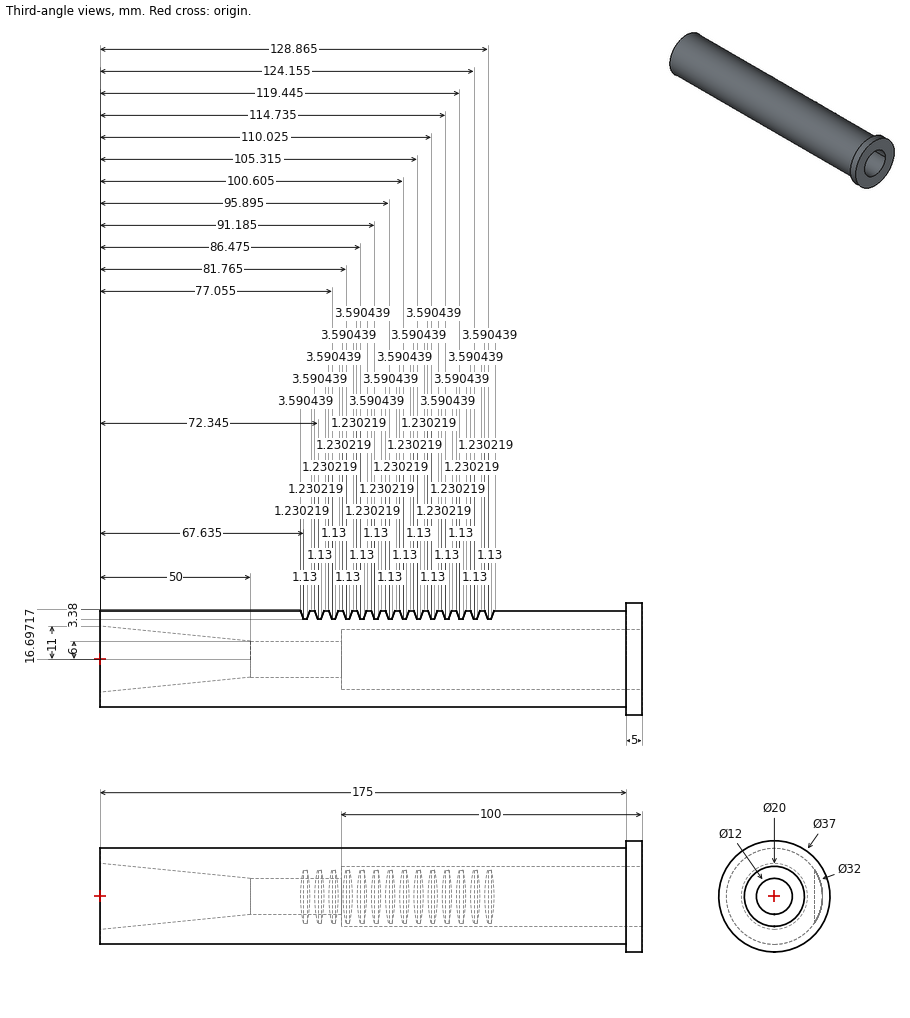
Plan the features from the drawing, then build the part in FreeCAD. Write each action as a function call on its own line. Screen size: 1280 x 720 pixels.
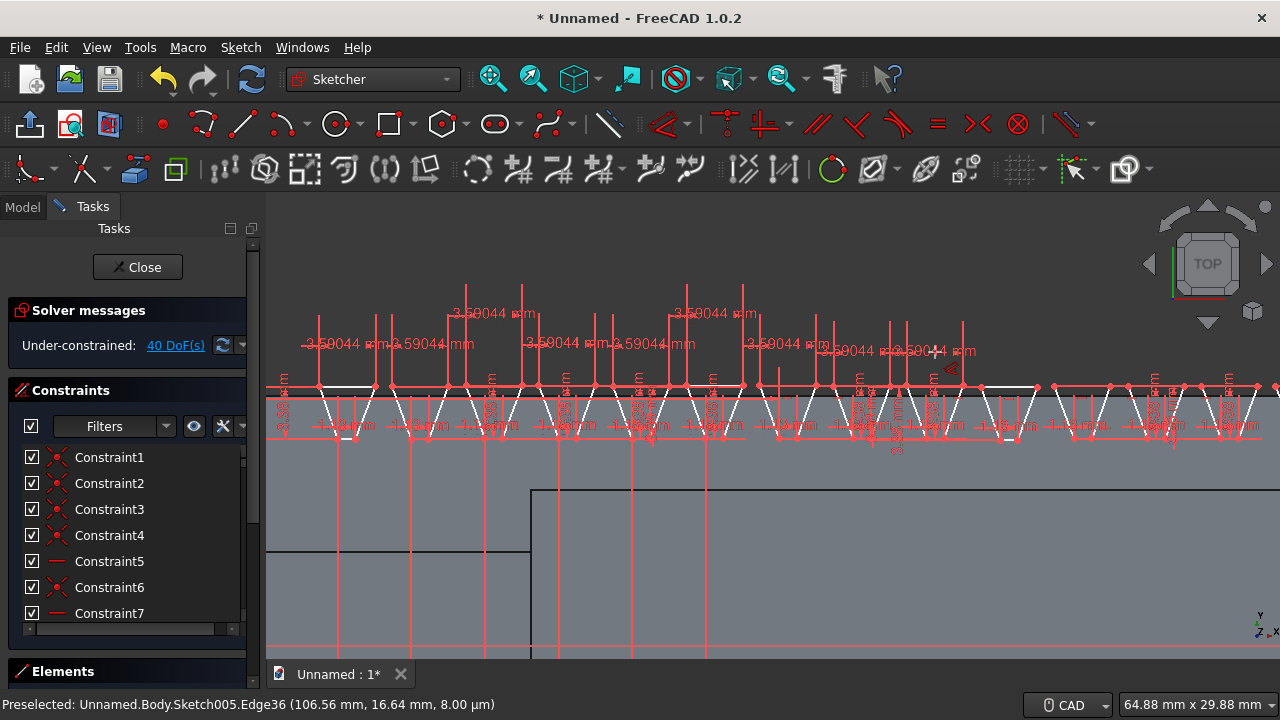
click(1020, 387)
click(1009, 353)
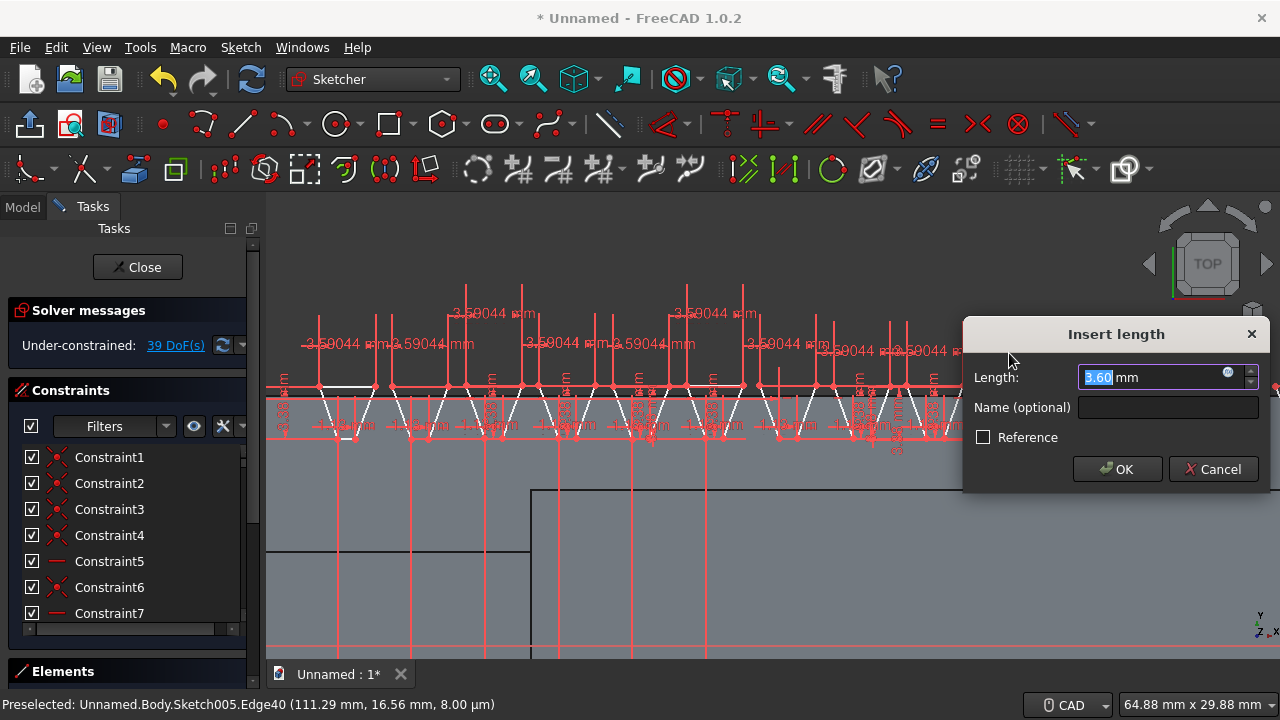
text(3.590439)
key(Return)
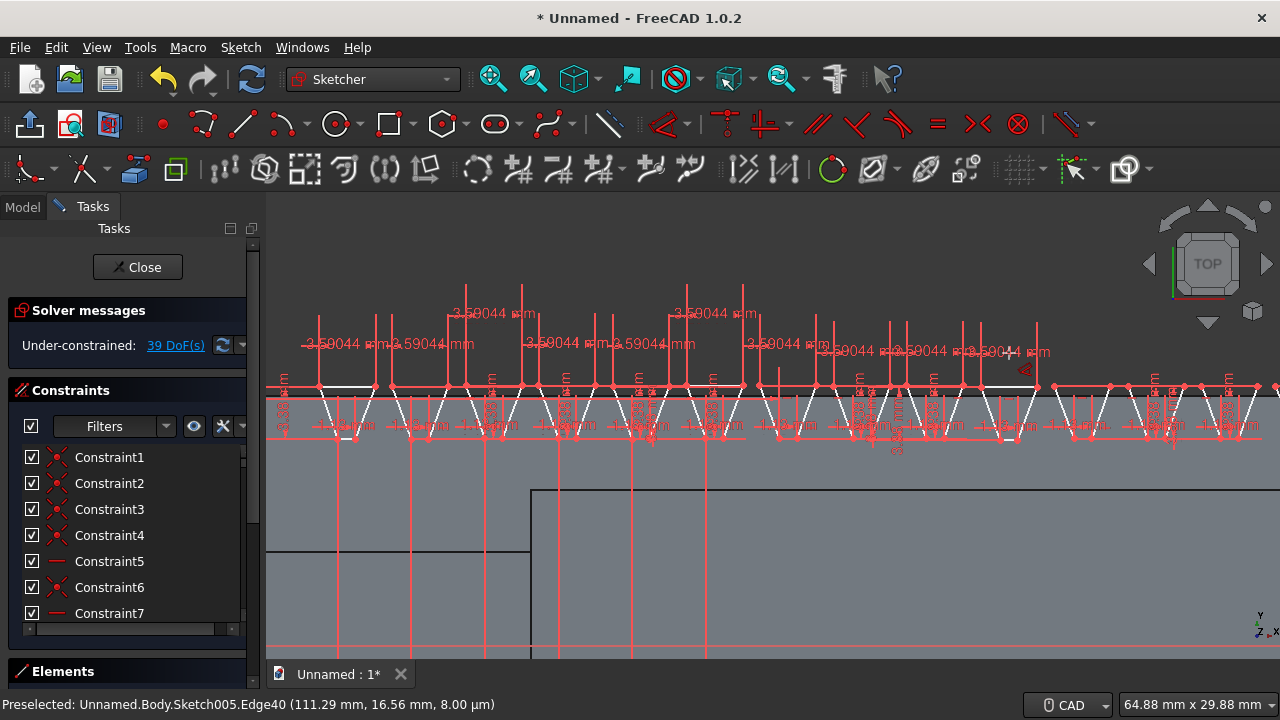
click(1094, 386)
click(1082, 352)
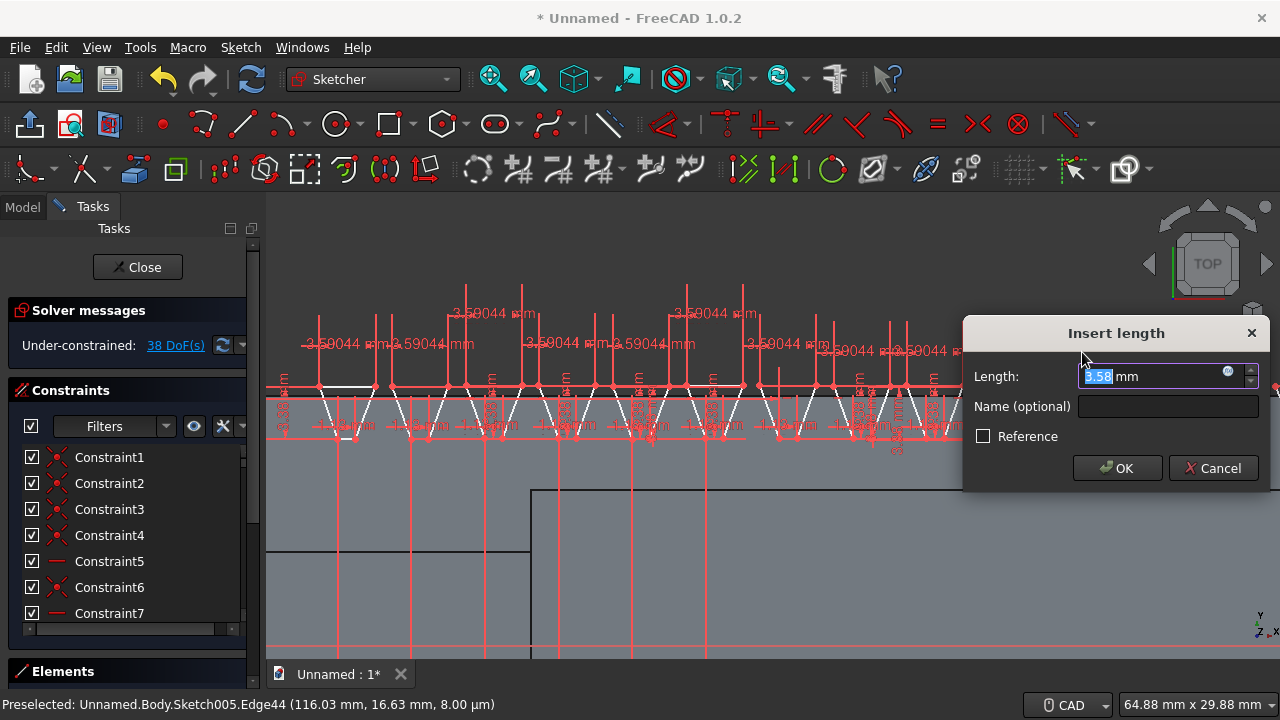
text(3.590439)
key(Return)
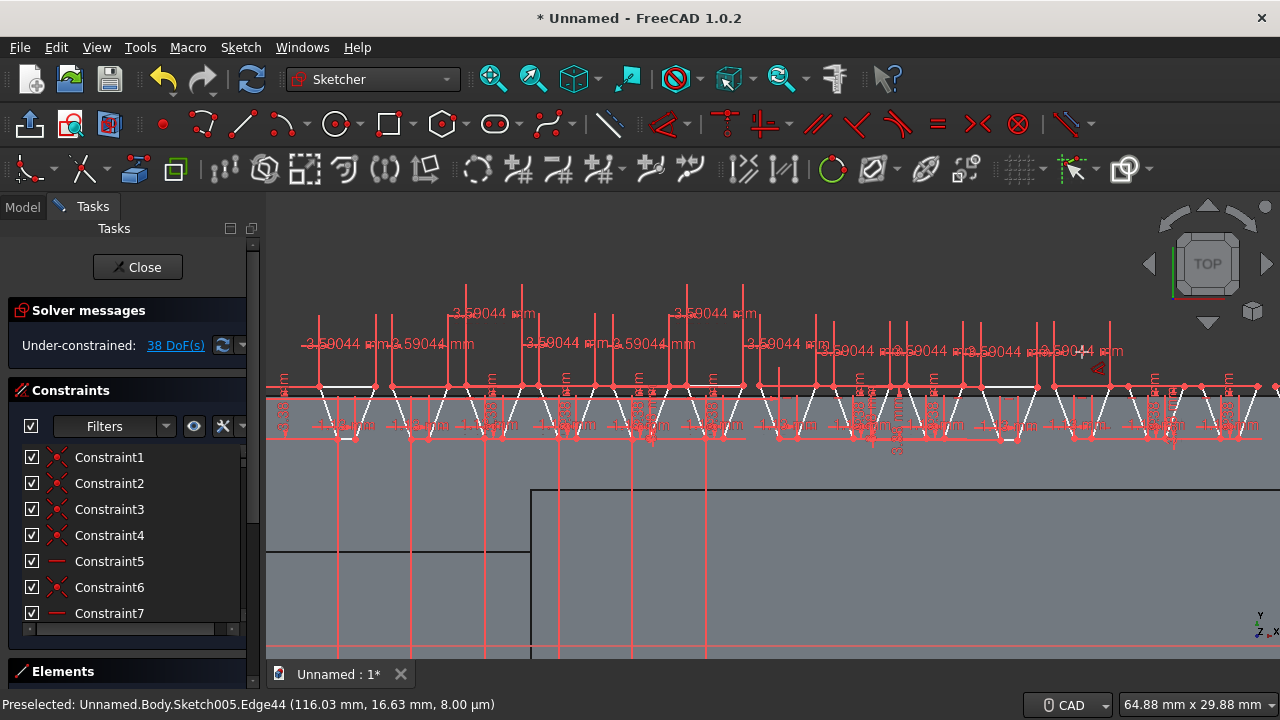
scroll(876, 387, down, 6)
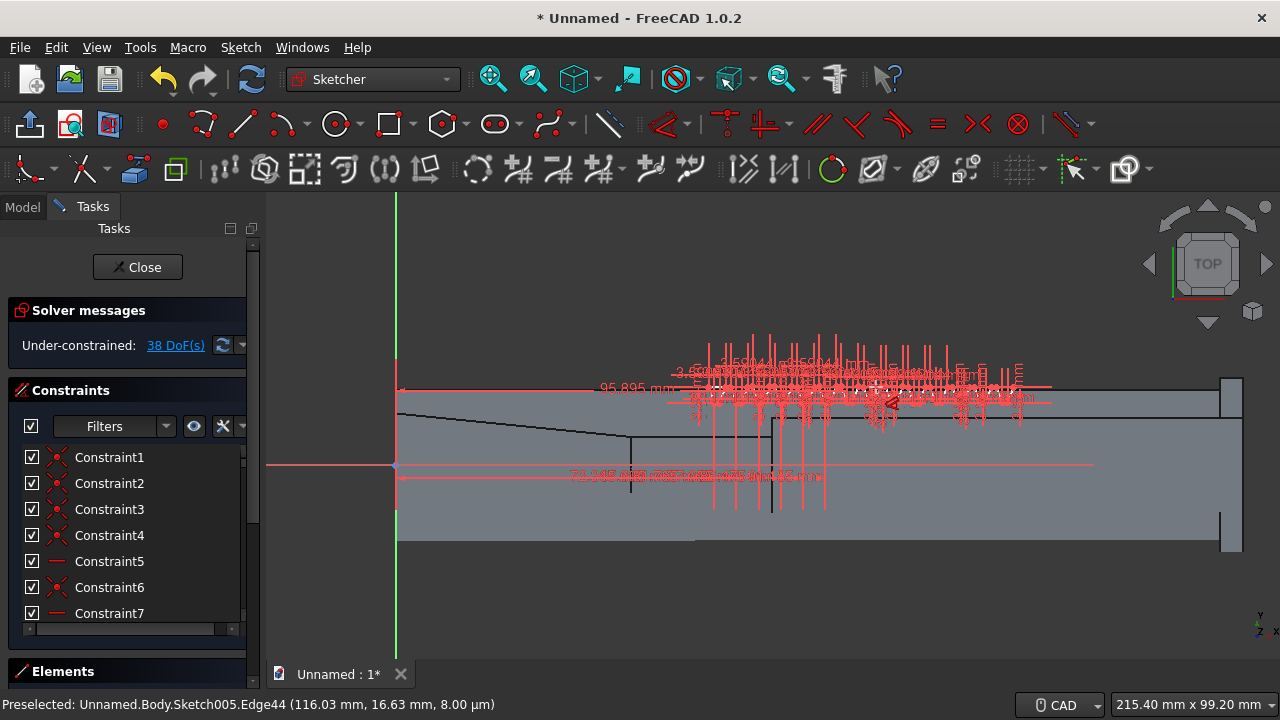
scroll(964, 387, up, 6)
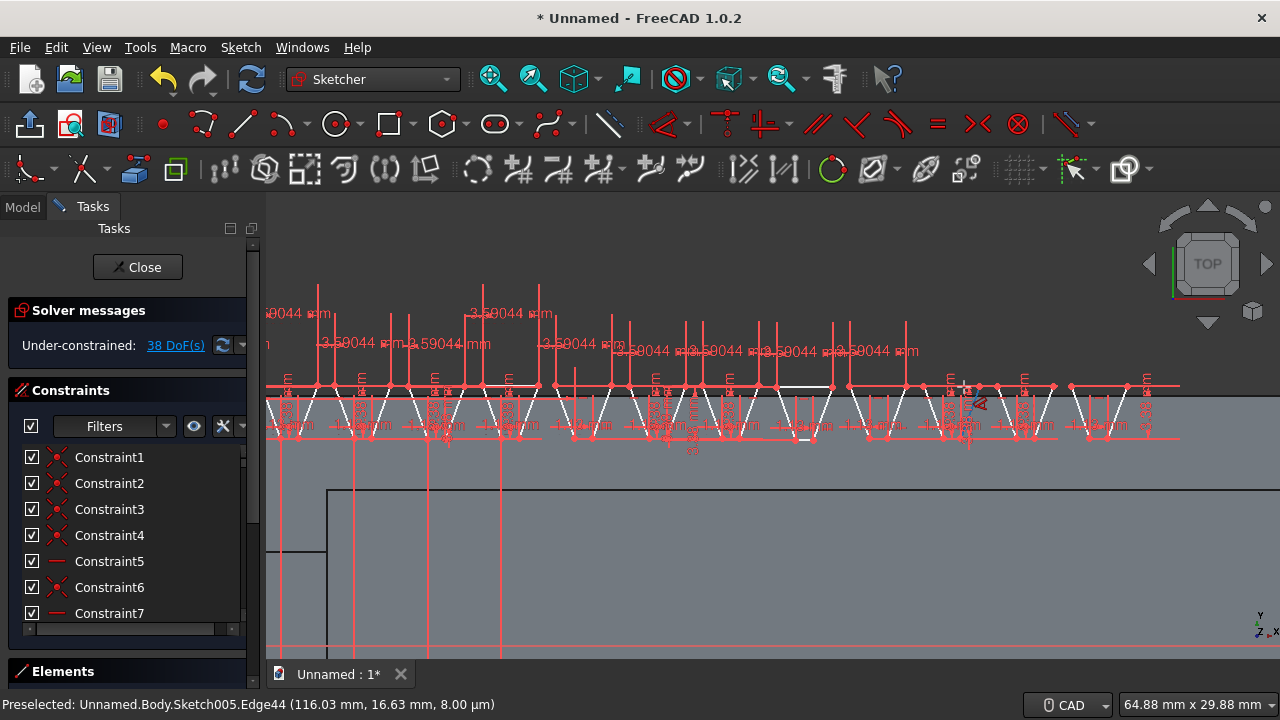
click(963, 386)
click(952, 352)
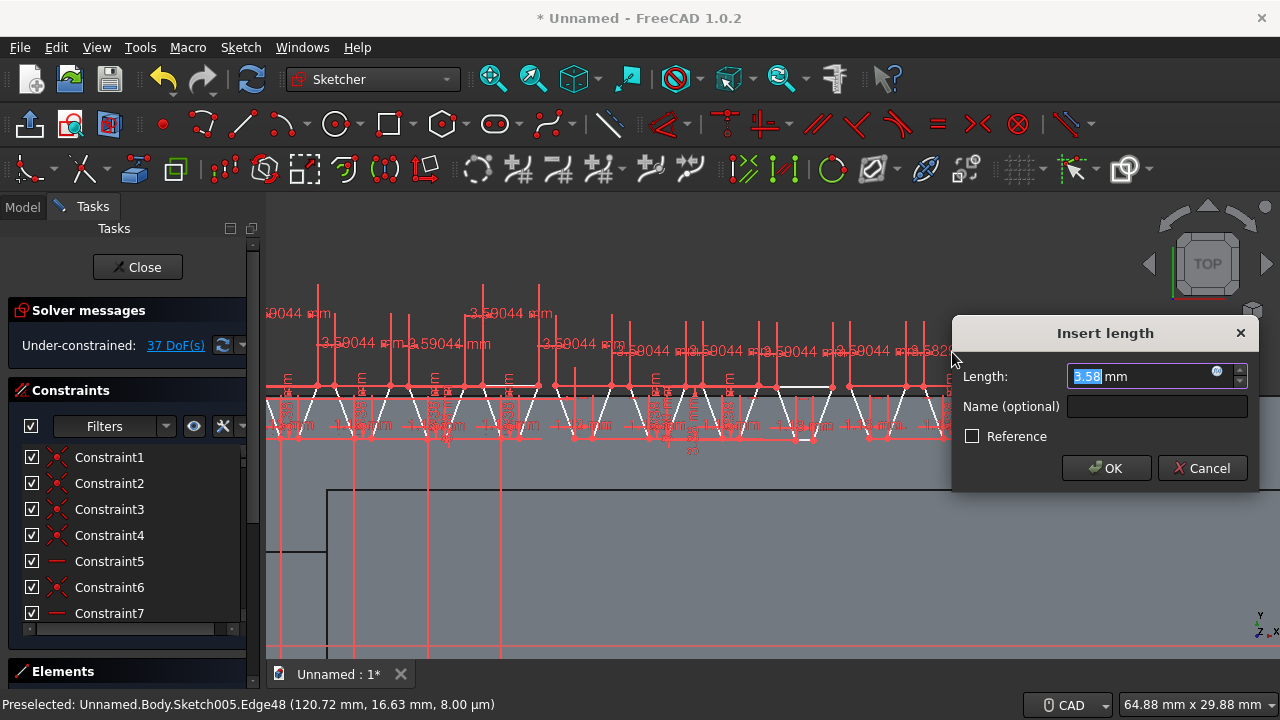
text(3.590439)
key(Return)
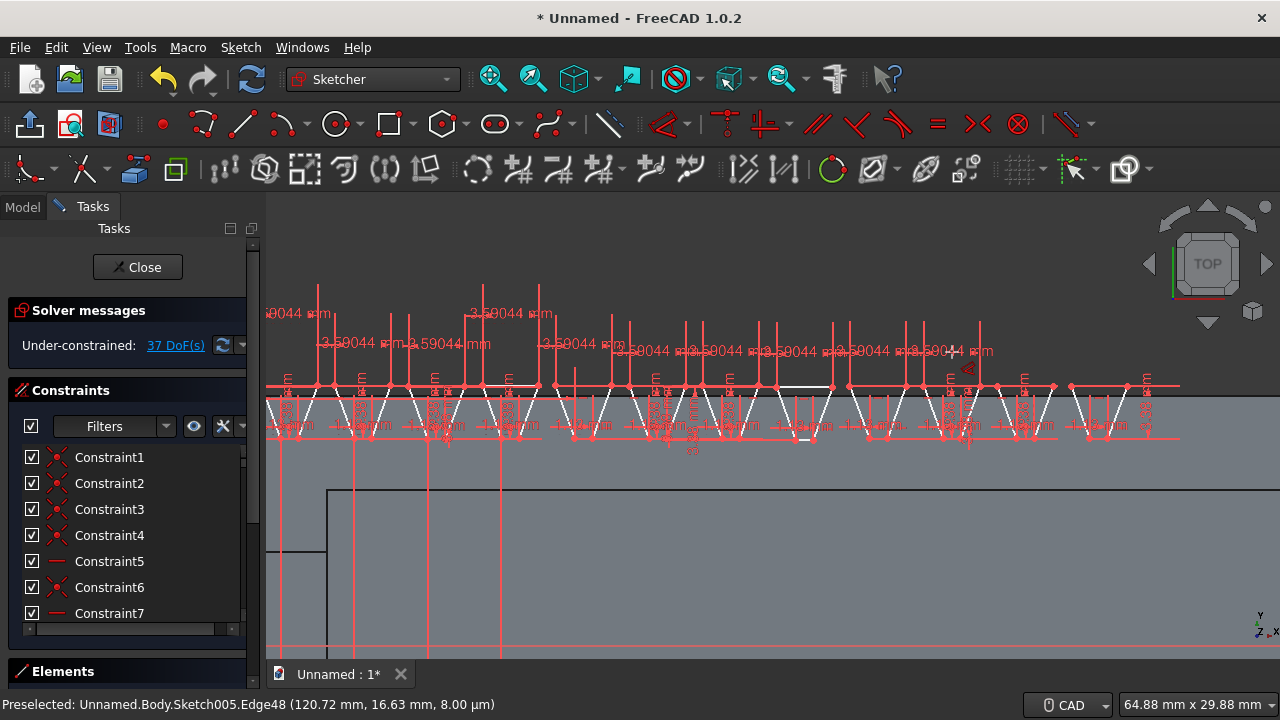
click(1037, 386)
click(1026, 352)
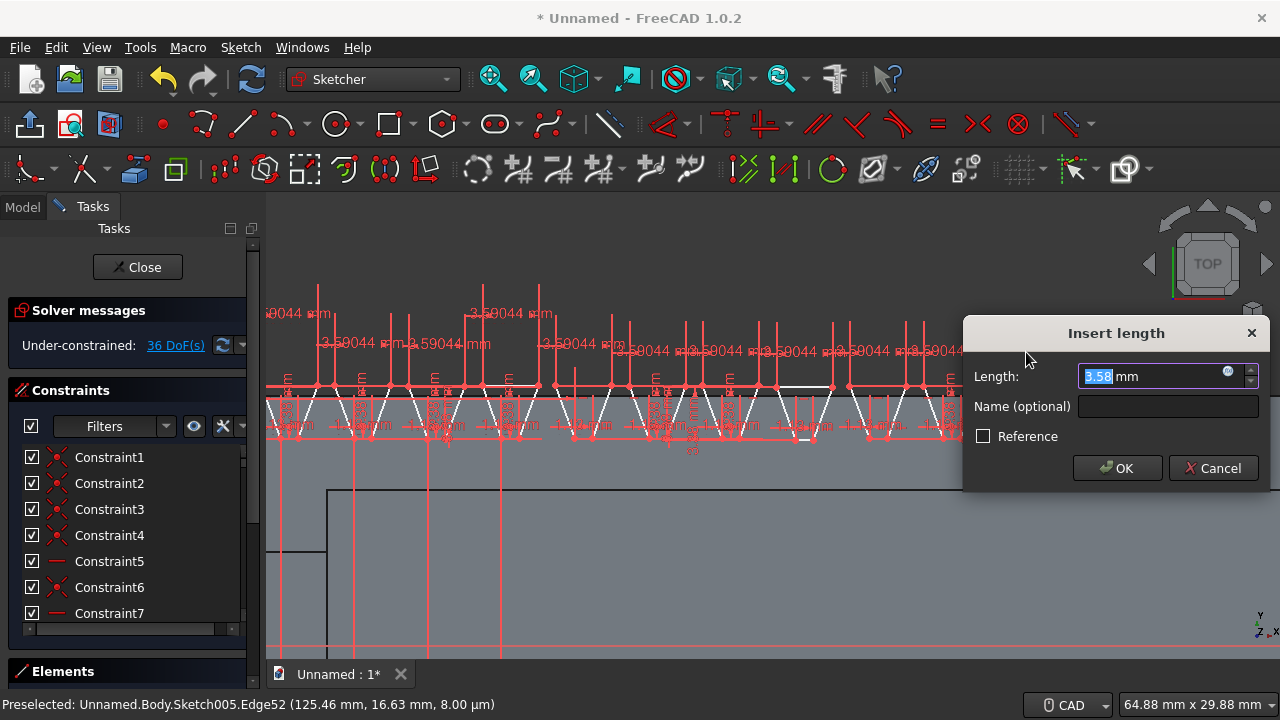
text(3.590439)
key(Return)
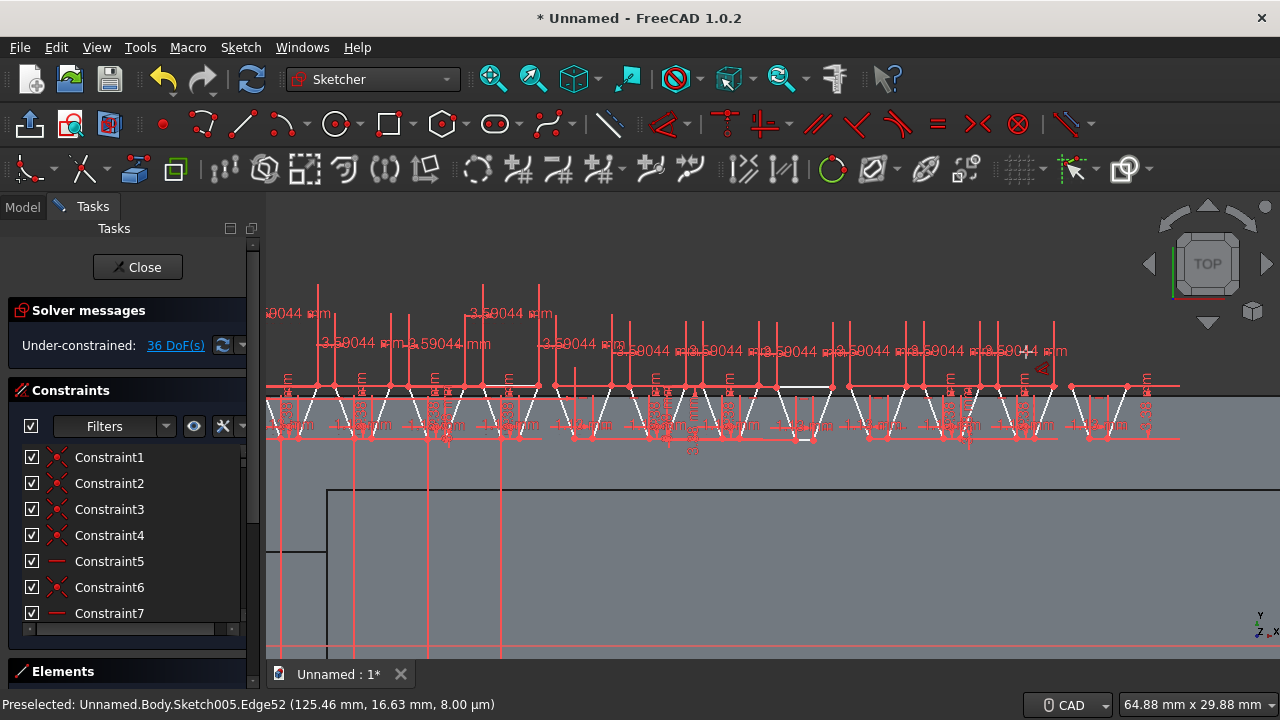
click(1111, 386)
click(1103, 352)